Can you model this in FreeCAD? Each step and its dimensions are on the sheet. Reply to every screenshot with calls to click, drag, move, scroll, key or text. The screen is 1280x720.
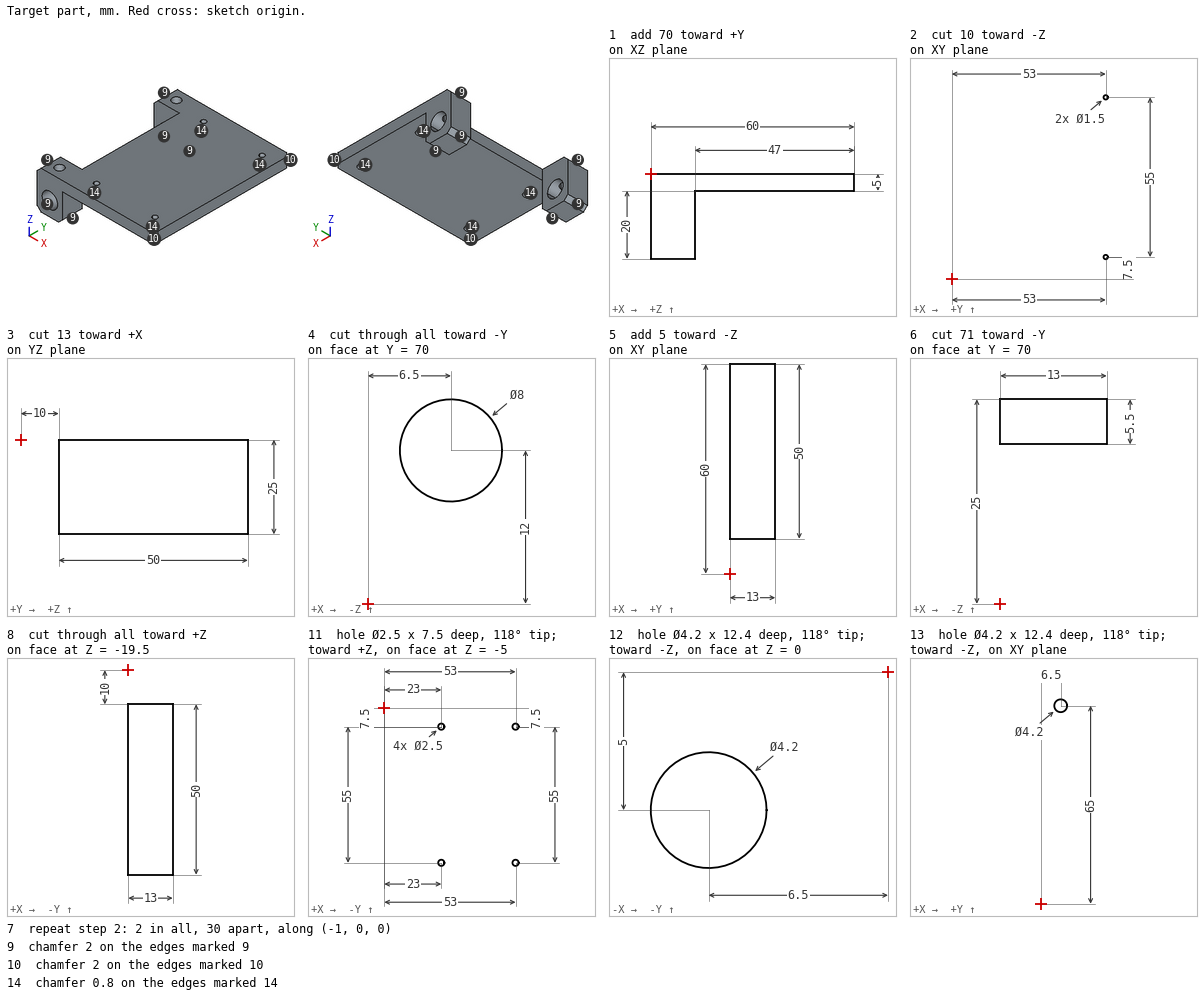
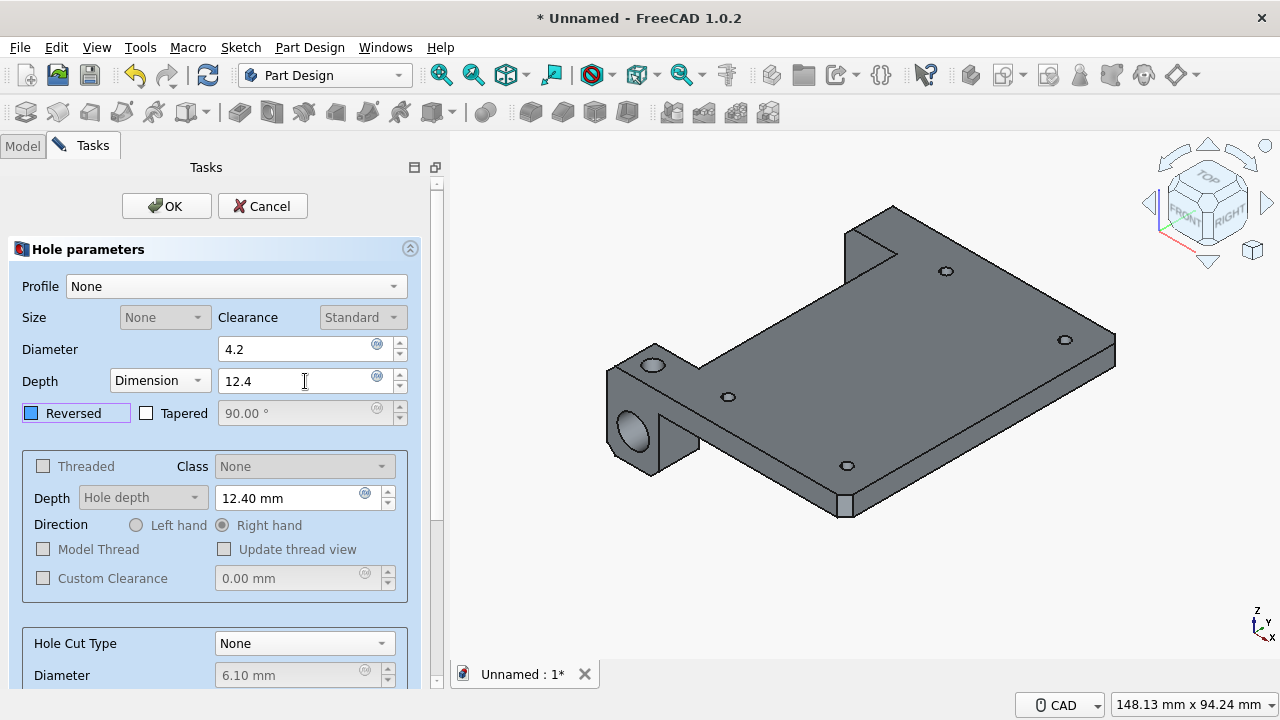
click(167, 206)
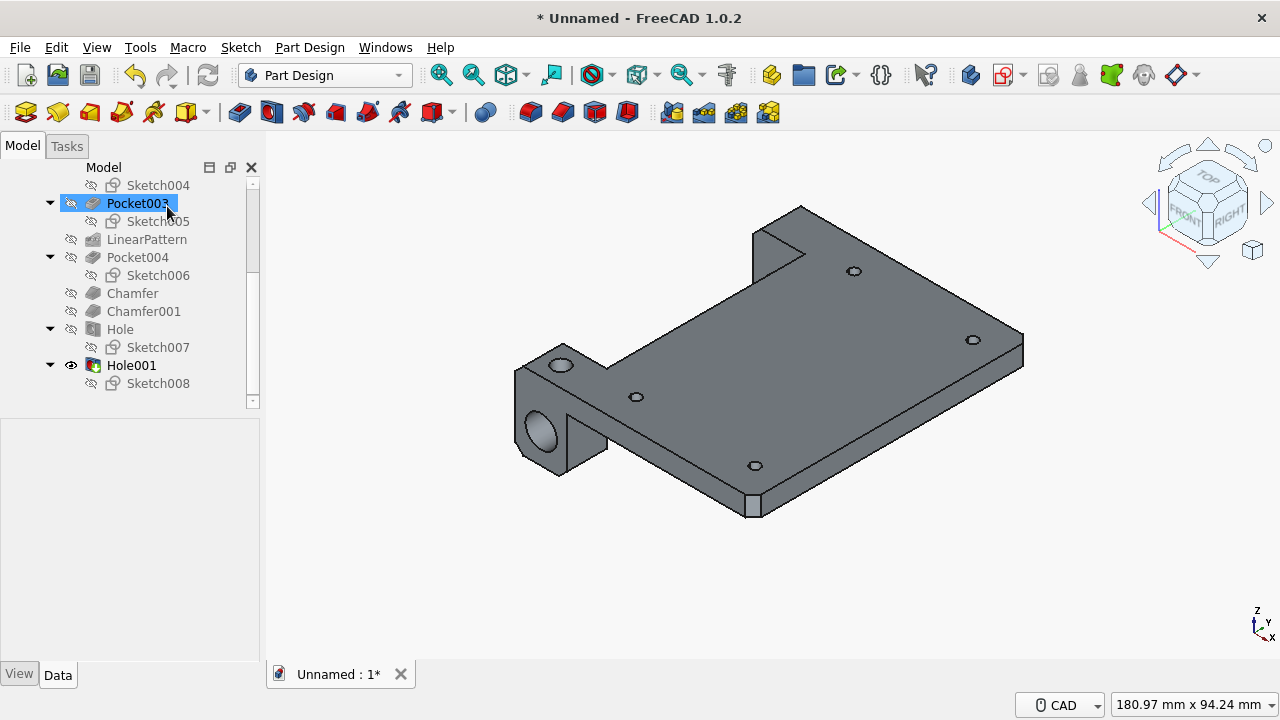
click(1004, 76)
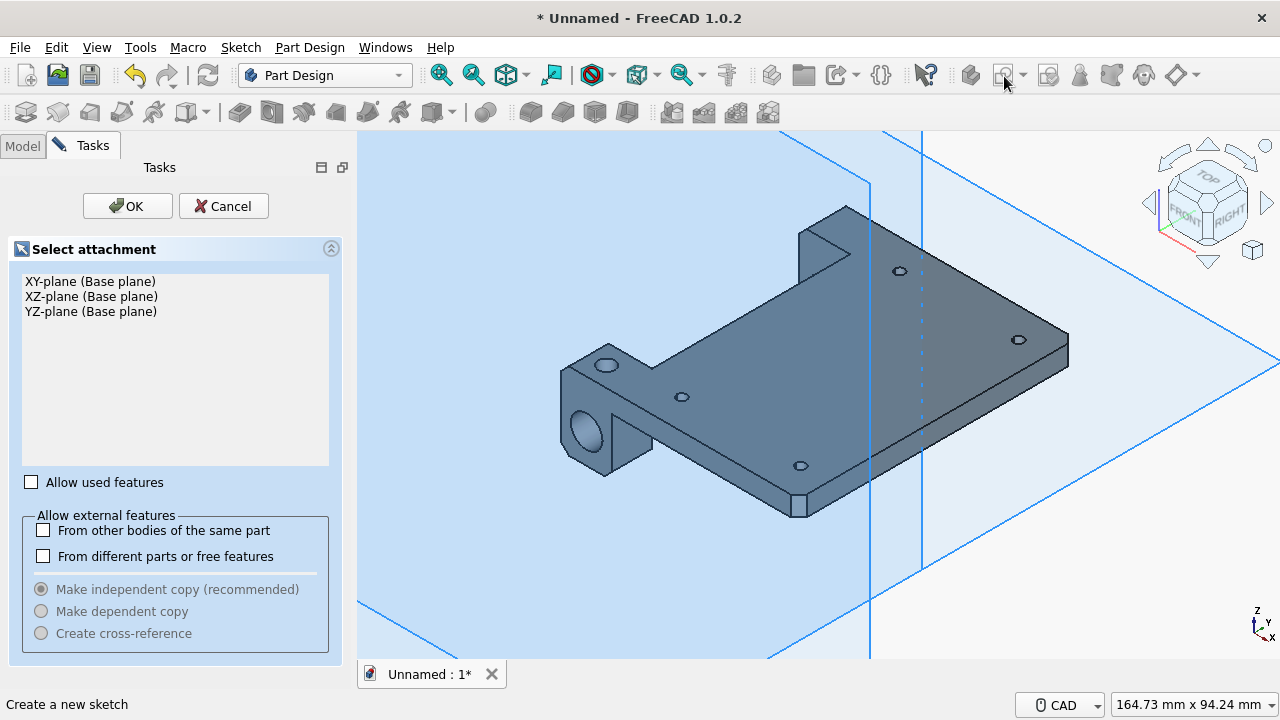
click(82, 282)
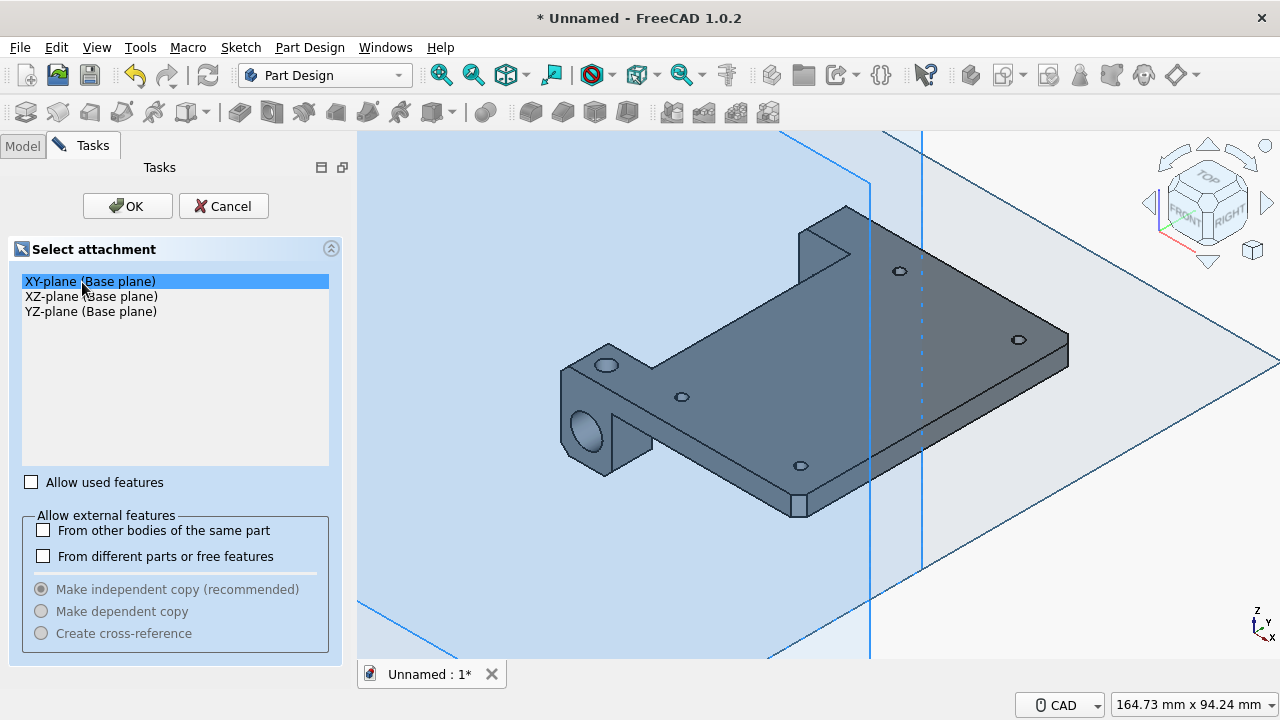
click(128, 206)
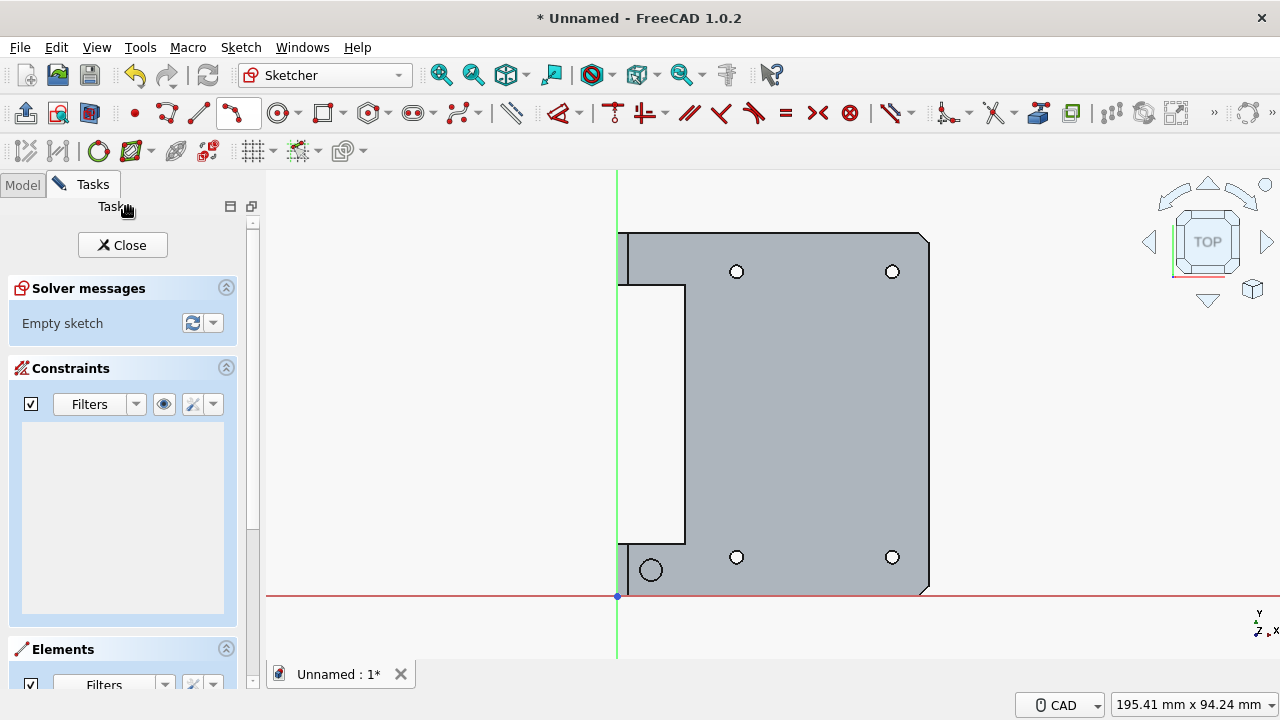
scroll(647, 246, up, 13)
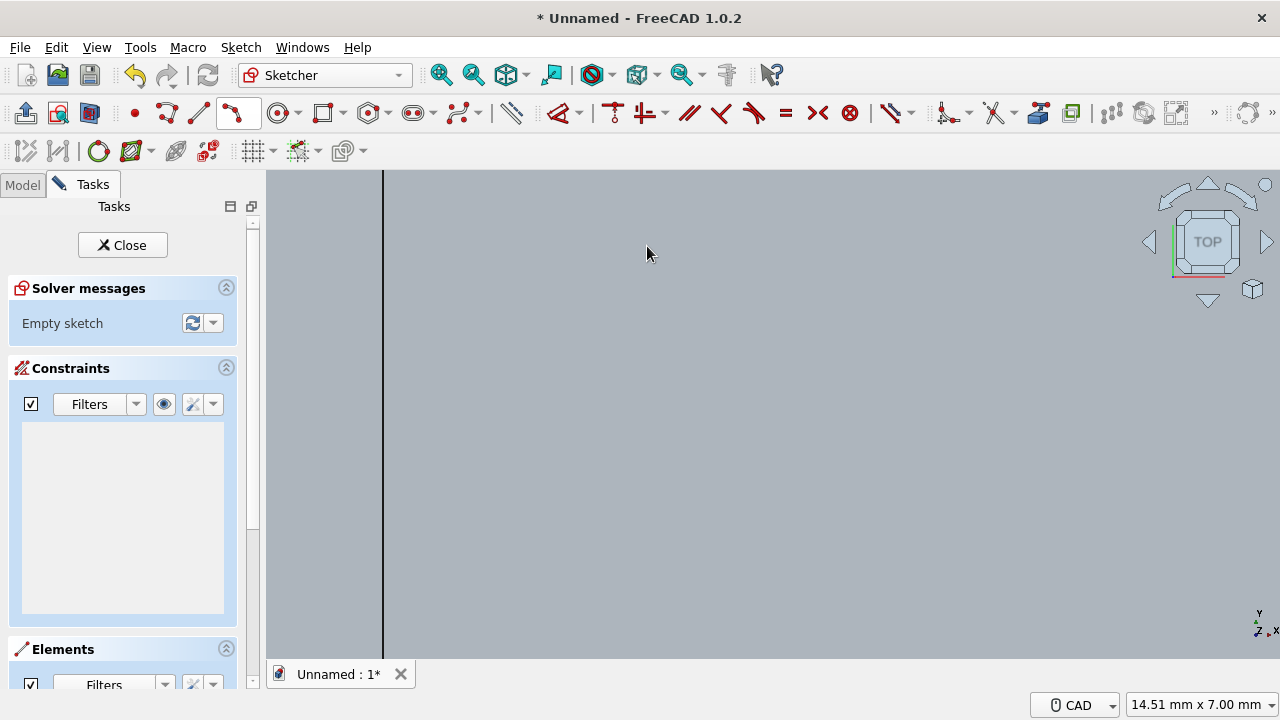
key(g)
key(c)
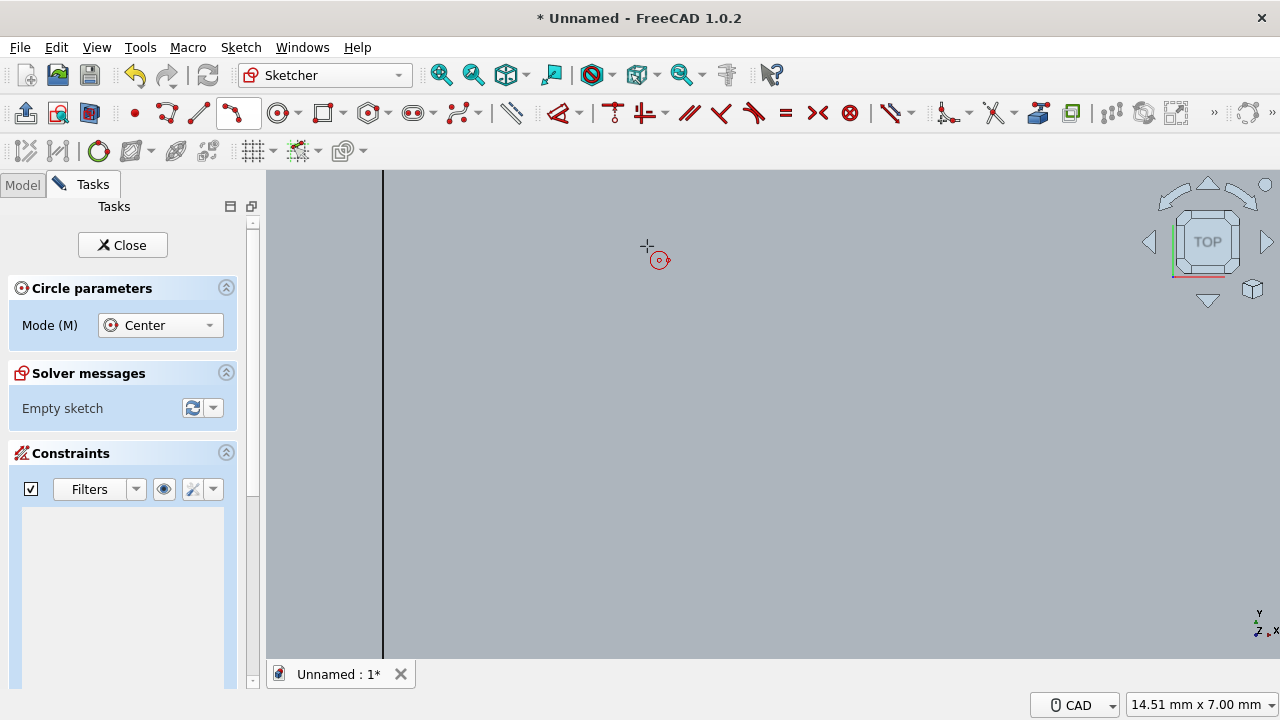
click(697, 417)
move(801, 313)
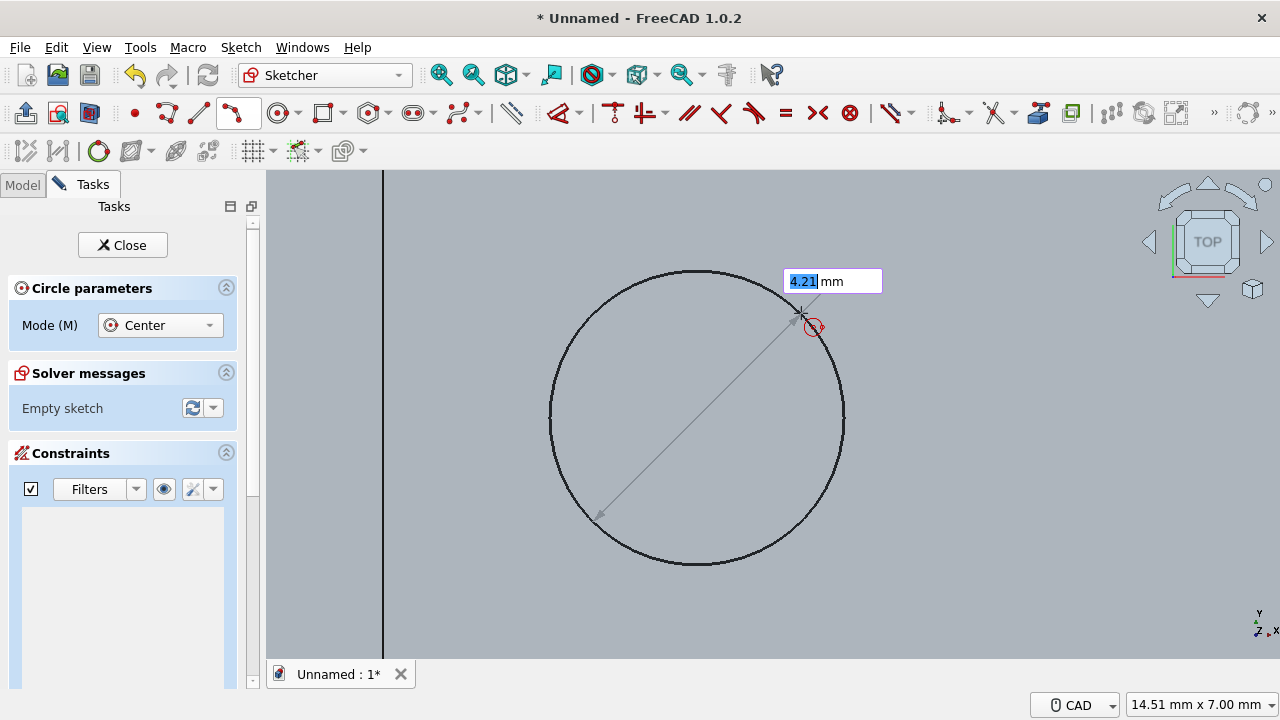
text(4.2)
key(Return)
key(Escape)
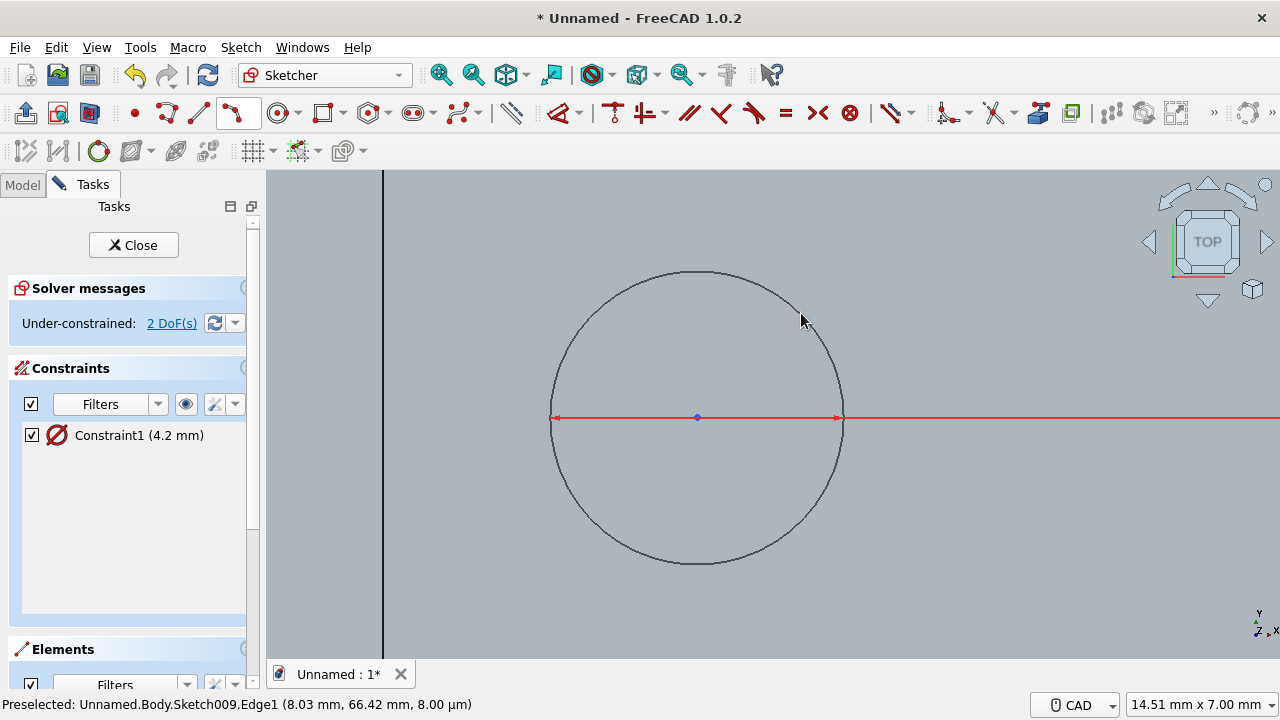
key(d)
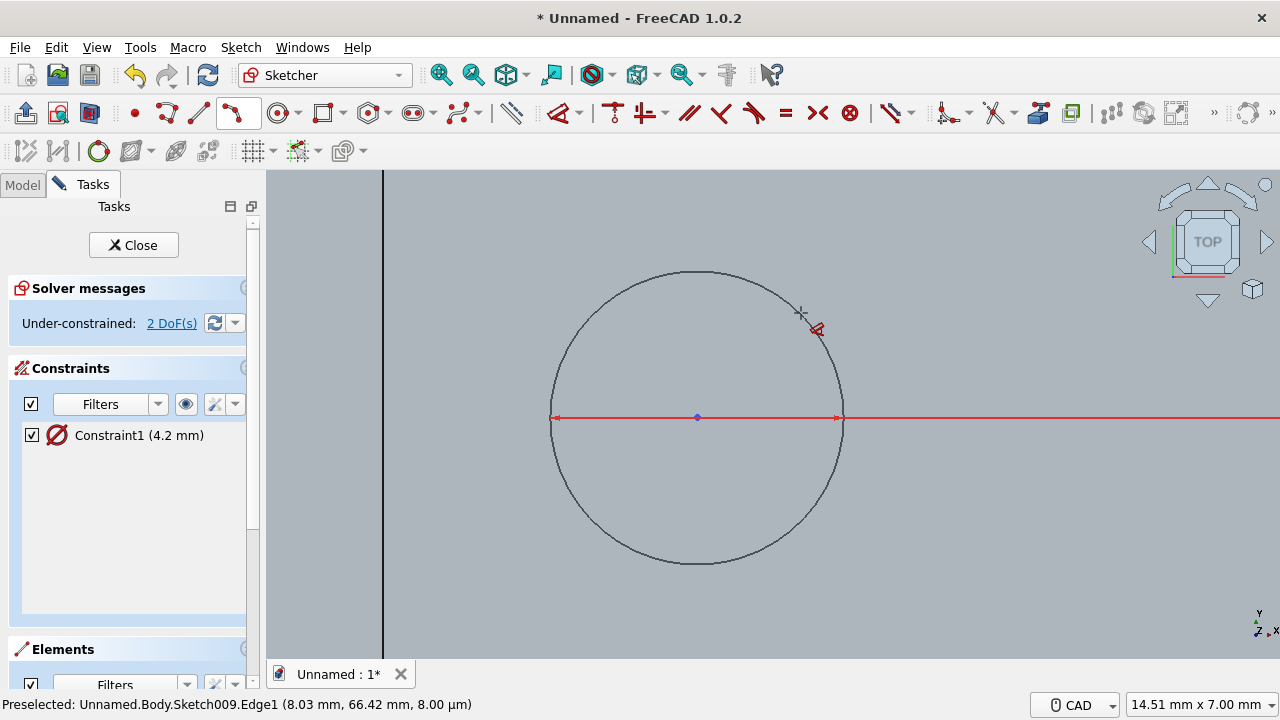
click(697, 418)
click(731, 524)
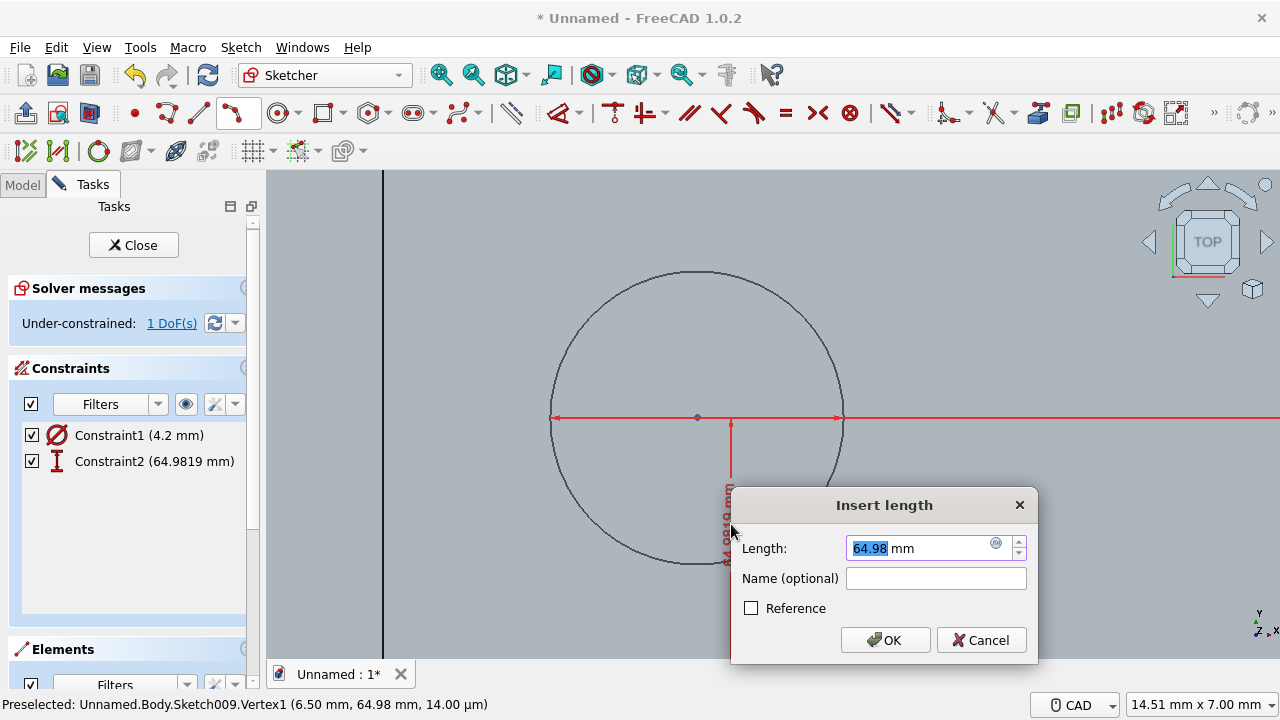
text(65)
key(Return)